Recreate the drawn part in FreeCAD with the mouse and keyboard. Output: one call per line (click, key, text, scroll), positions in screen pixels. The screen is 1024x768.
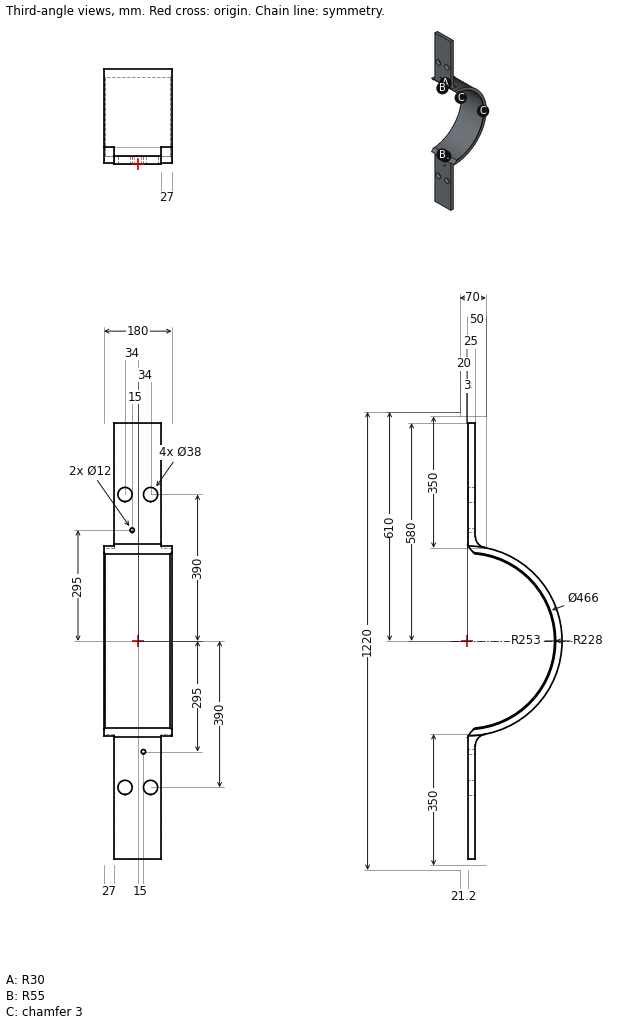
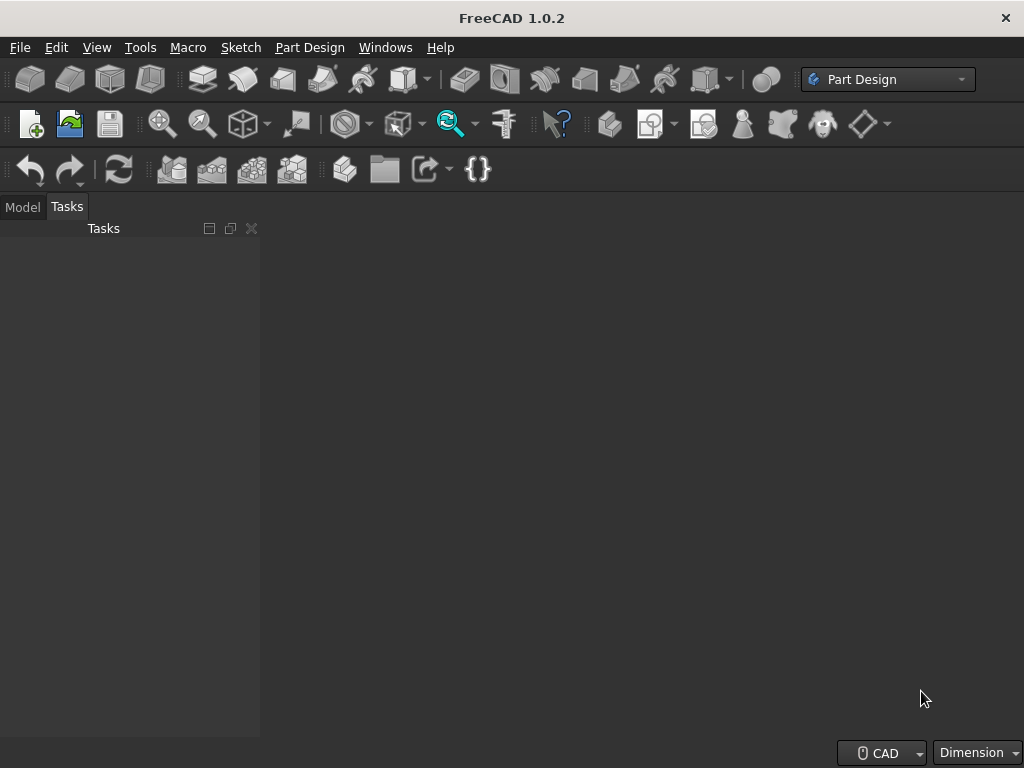
click(30, 124)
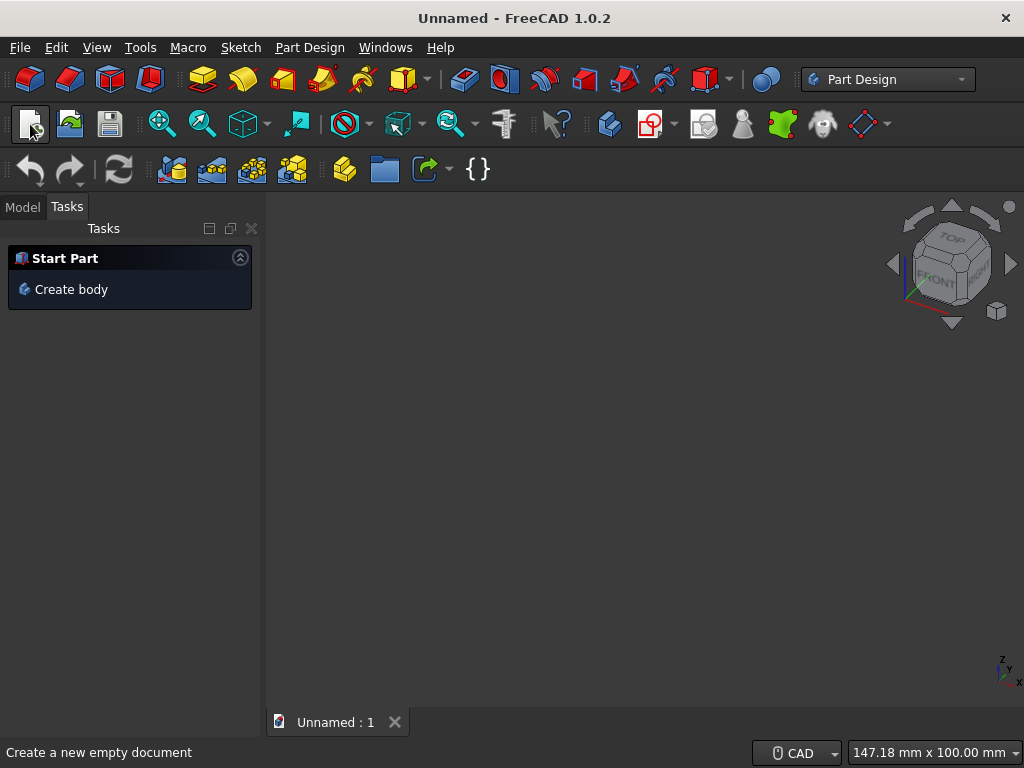
click(650, 124)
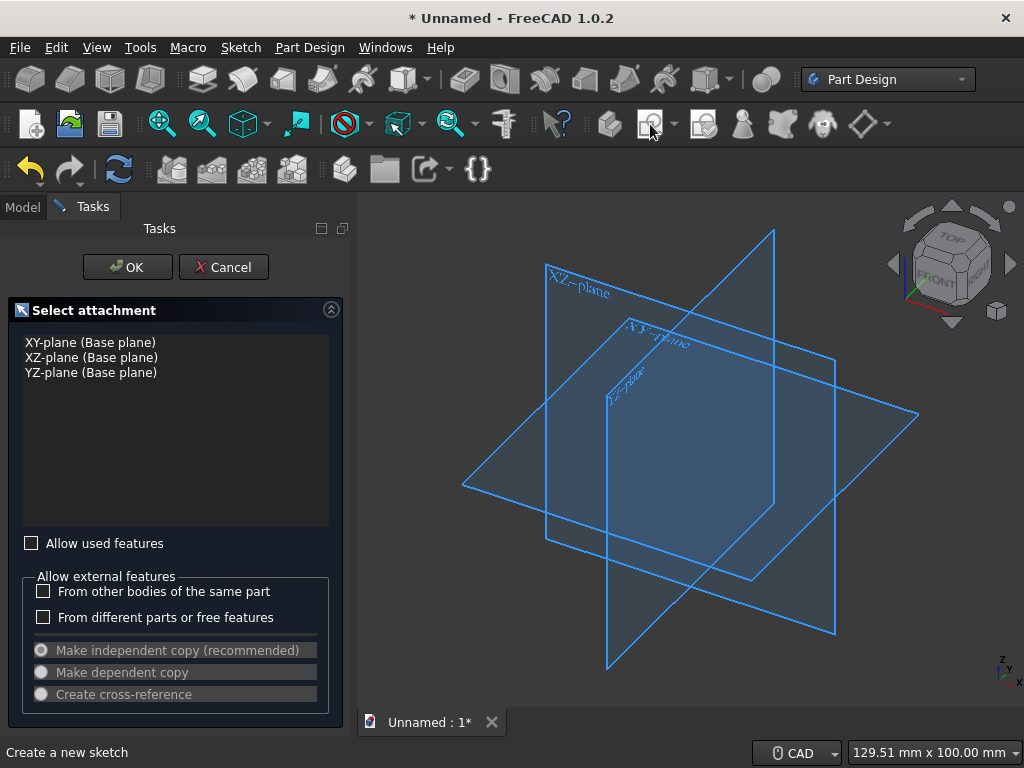
click(82, 372)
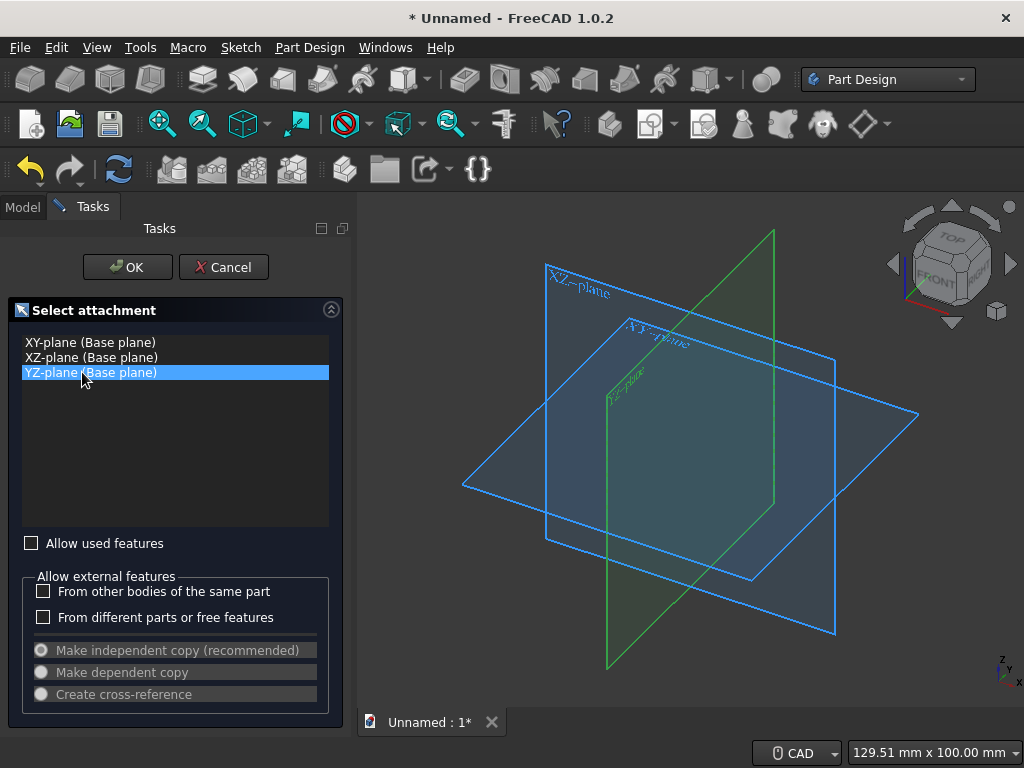
click(128, 267)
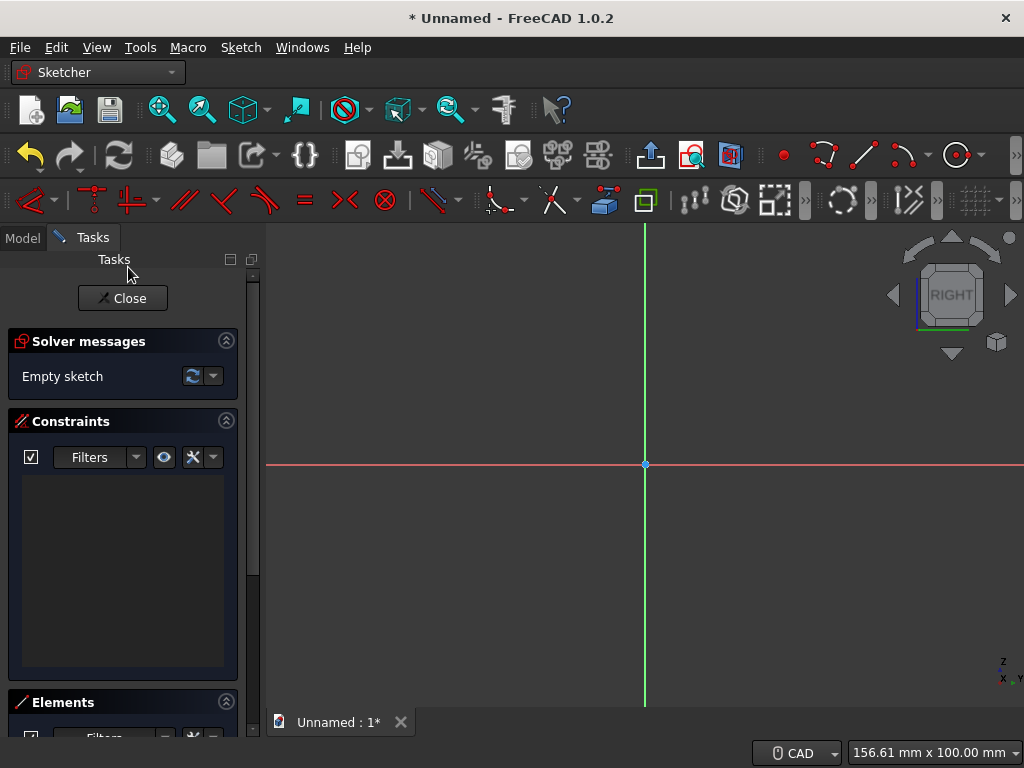
scroll(541, 465, down, 15)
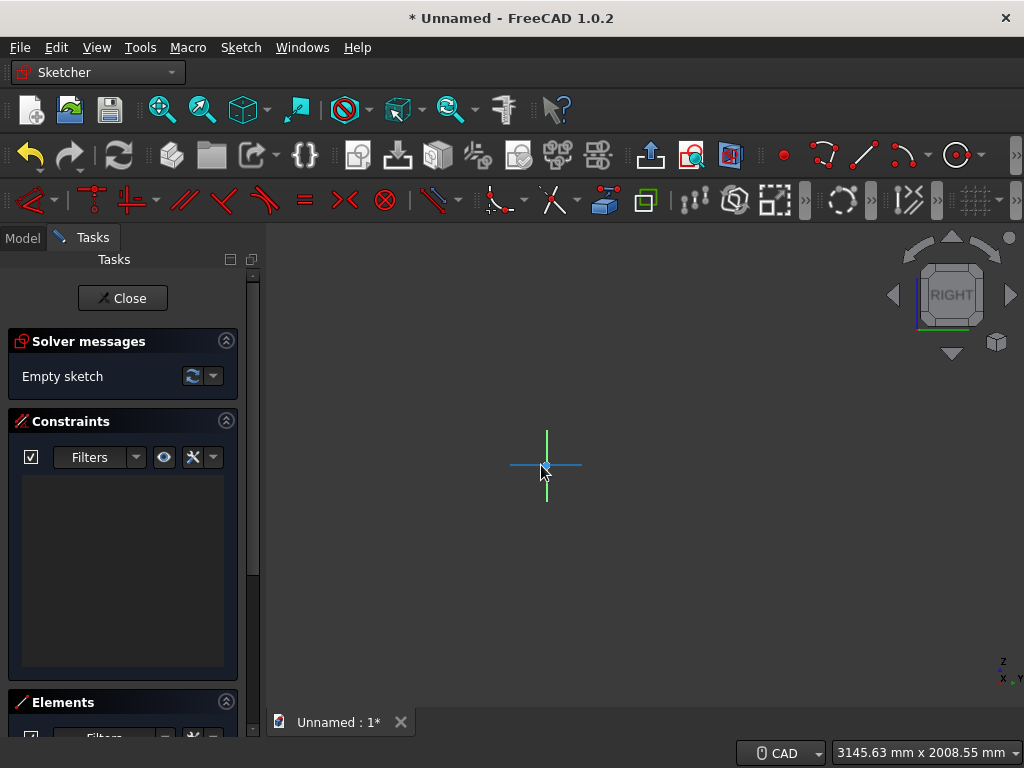
click(824, 156)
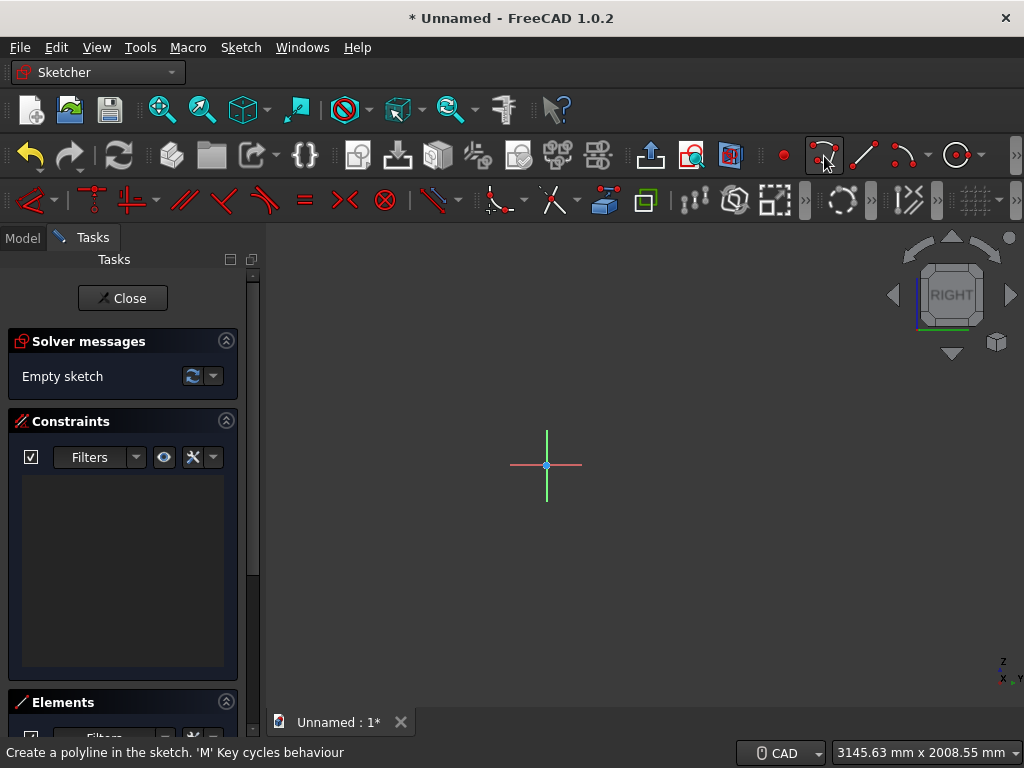
scroll(552, 405, up, 6)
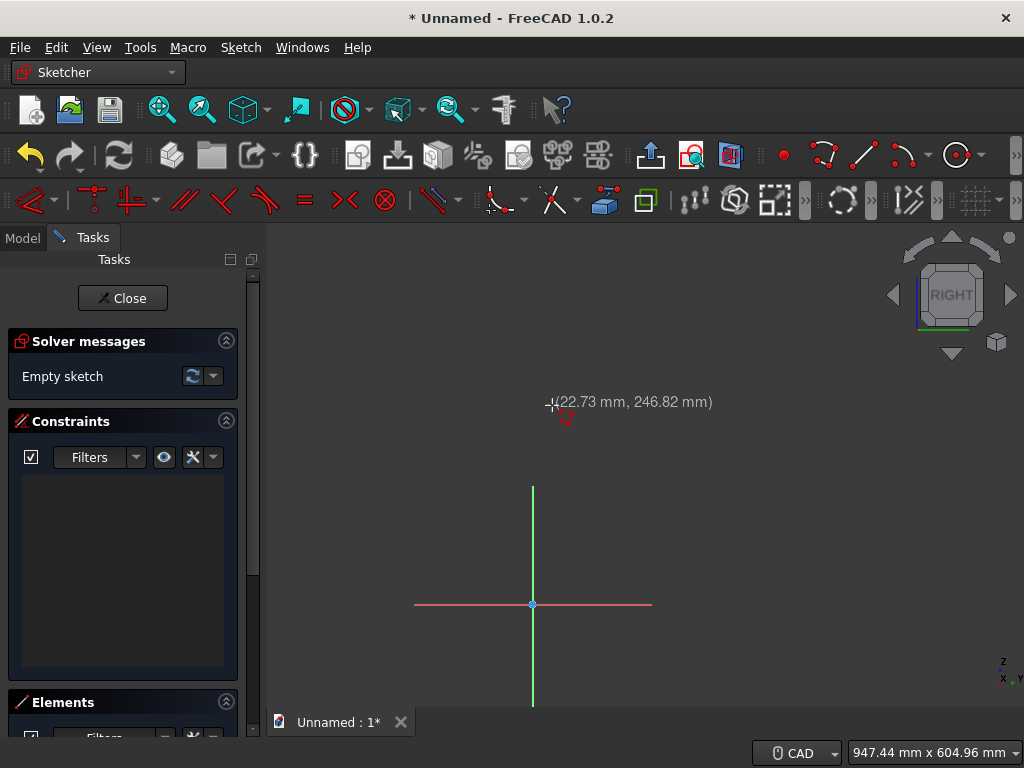
click(551, 403)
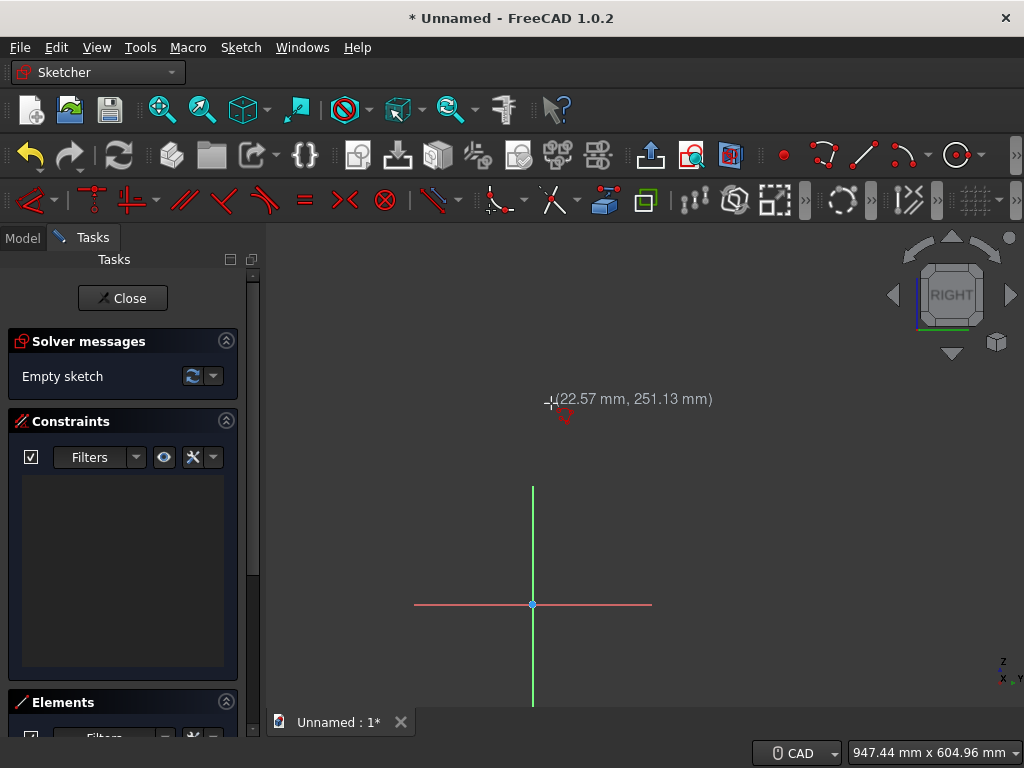
scroll(552, 405, down, 6)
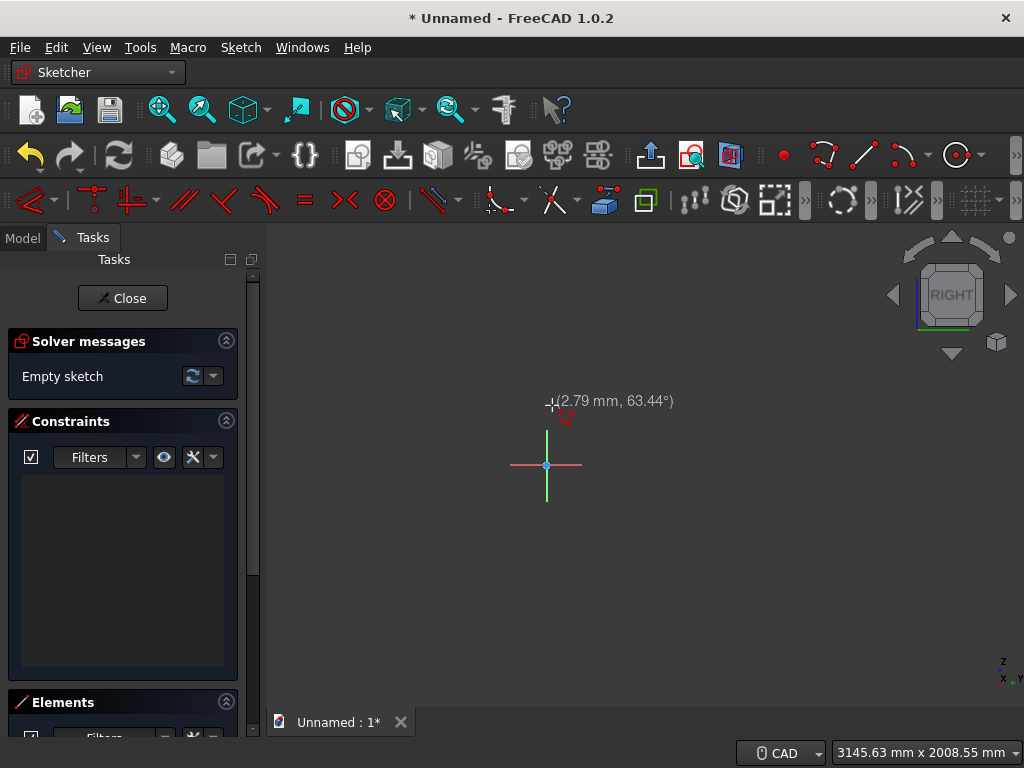
scroll(552, 326, up, 6)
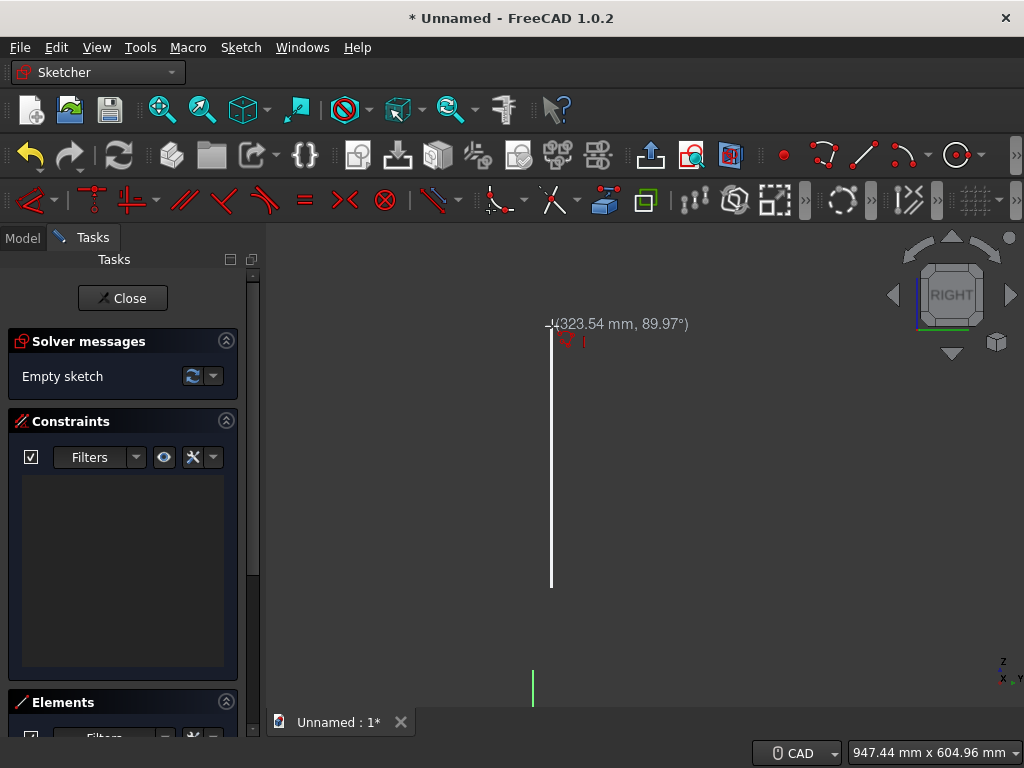
click(551, 325)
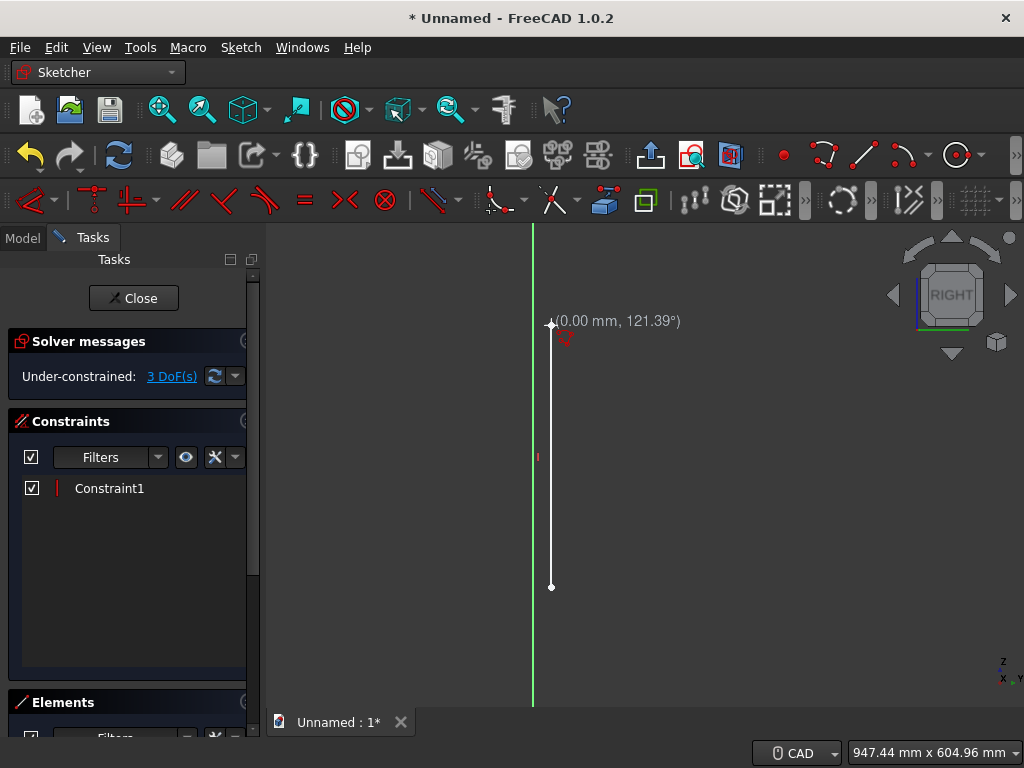
scroll(531, 325, up, 10)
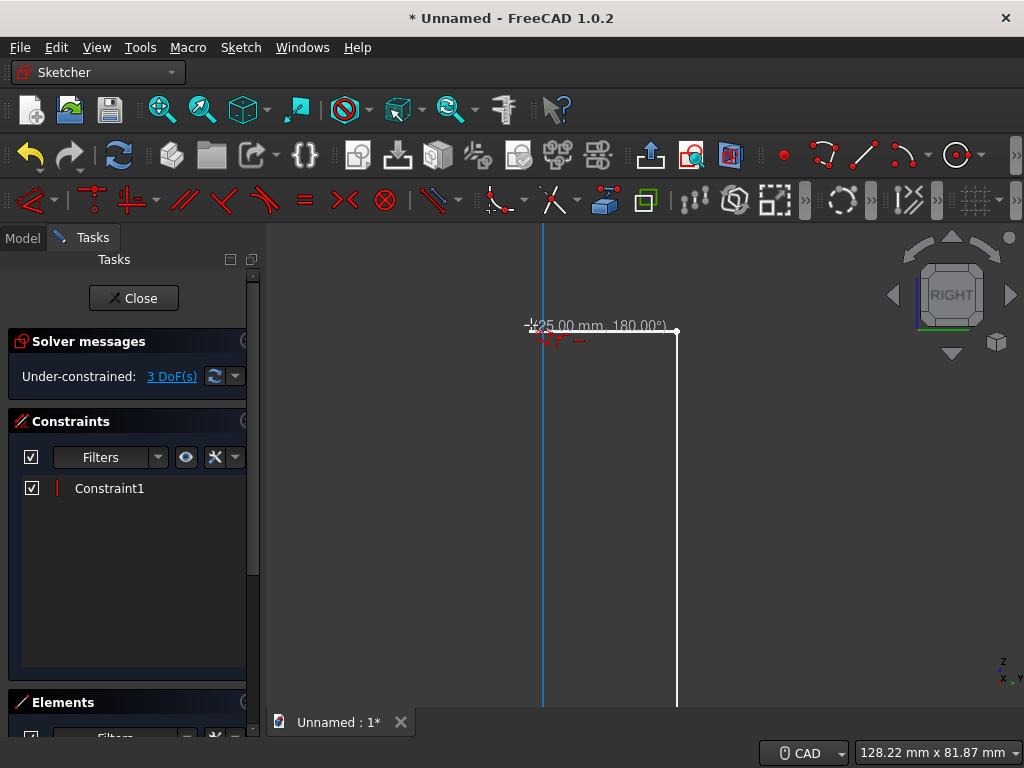
click(525, 324)